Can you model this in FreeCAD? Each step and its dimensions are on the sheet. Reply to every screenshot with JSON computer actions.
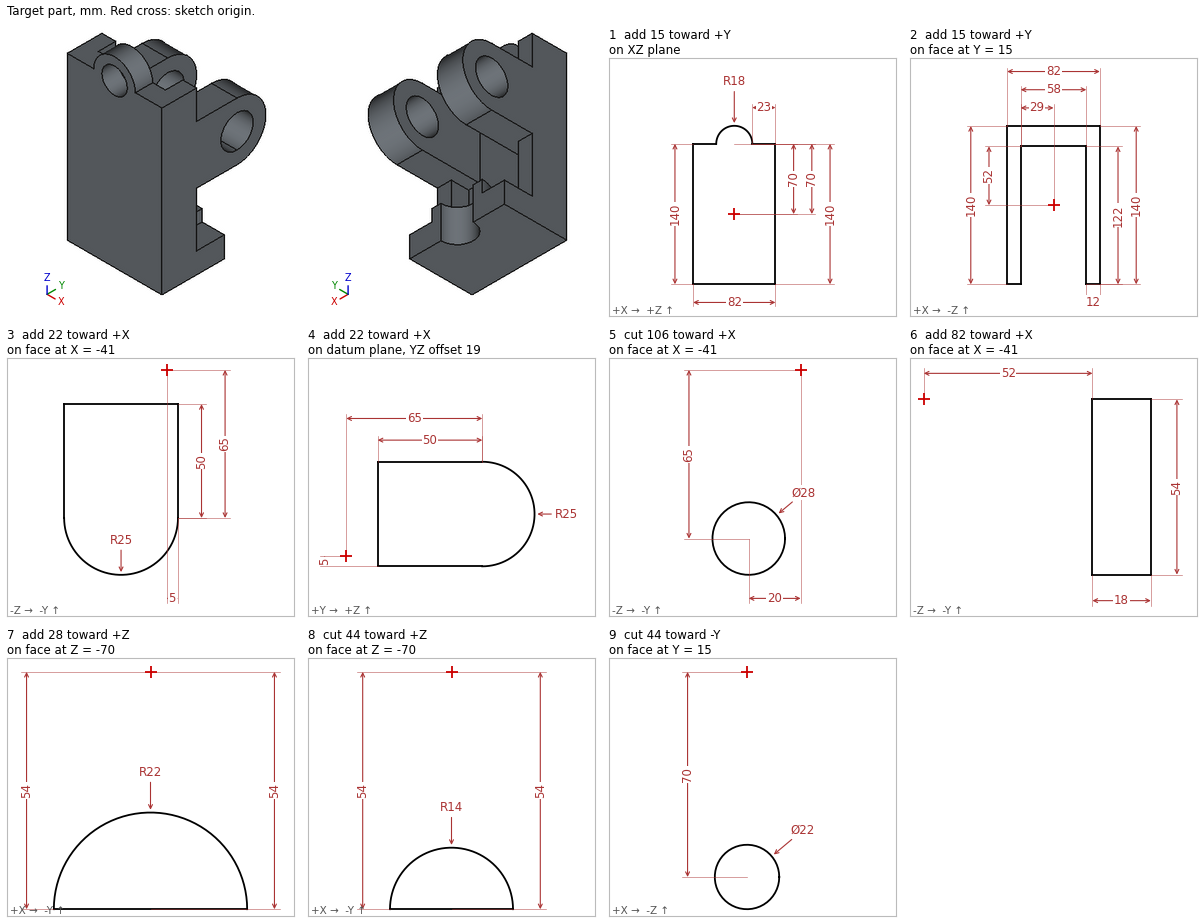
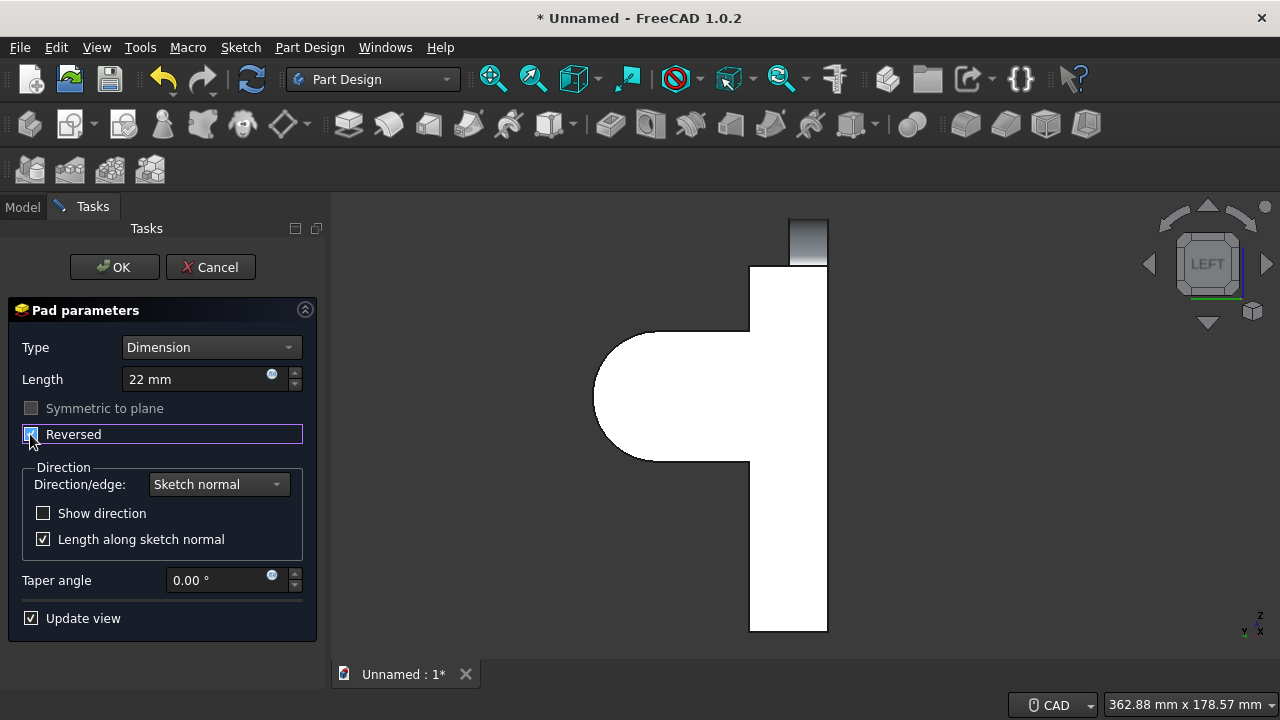
{"action": "left_click", "coordinate": [115, 267]}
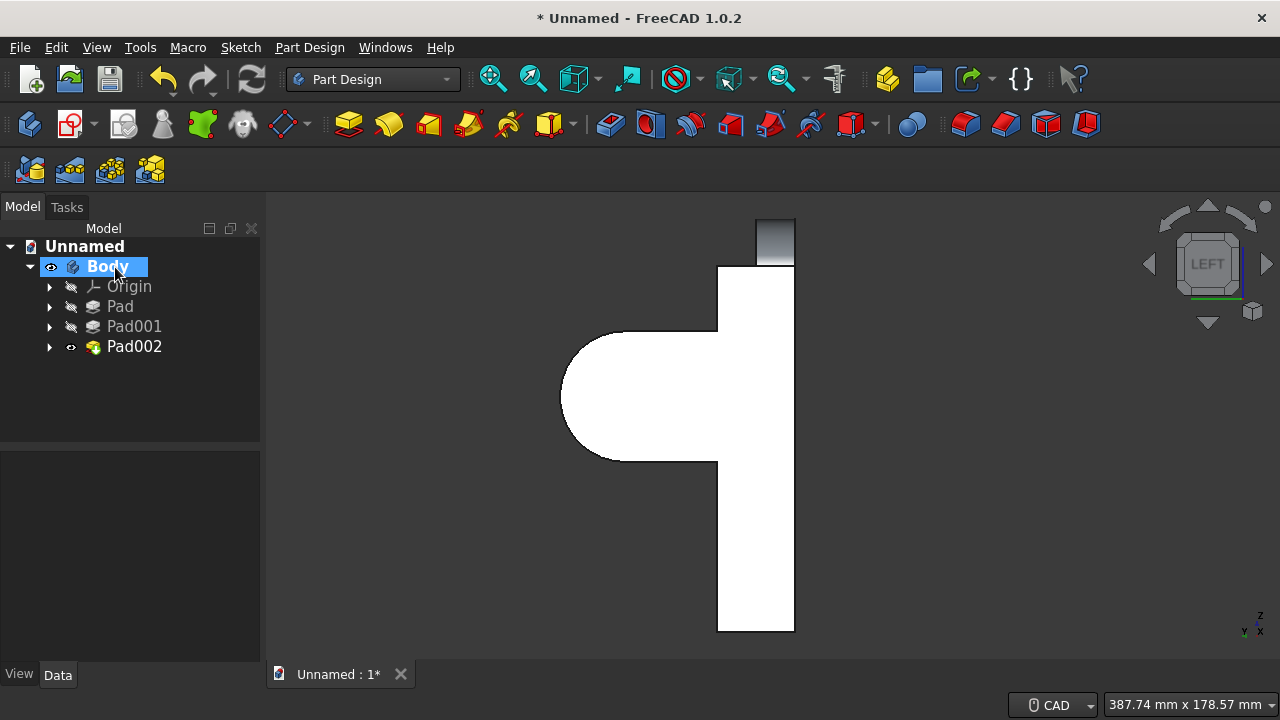
{"action": "left_click", "coordinate": [50, 287]}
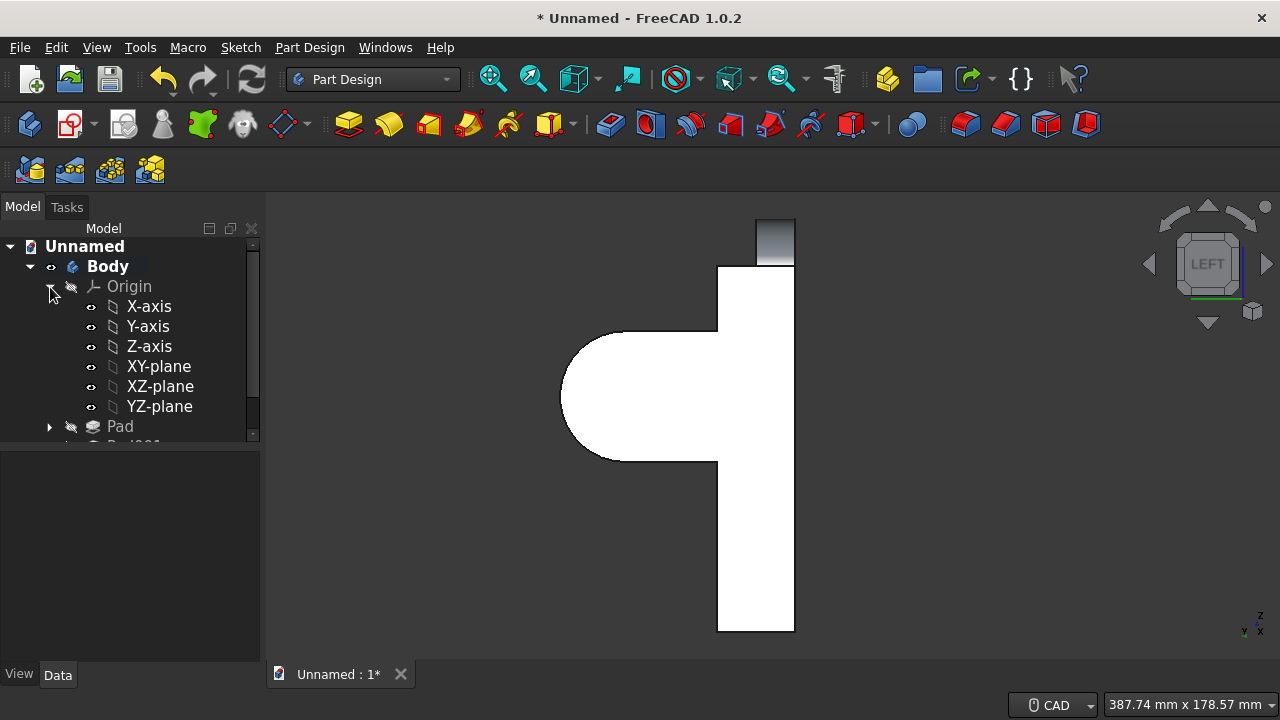
{"action": "left_click", "coordinate": [136, 407]}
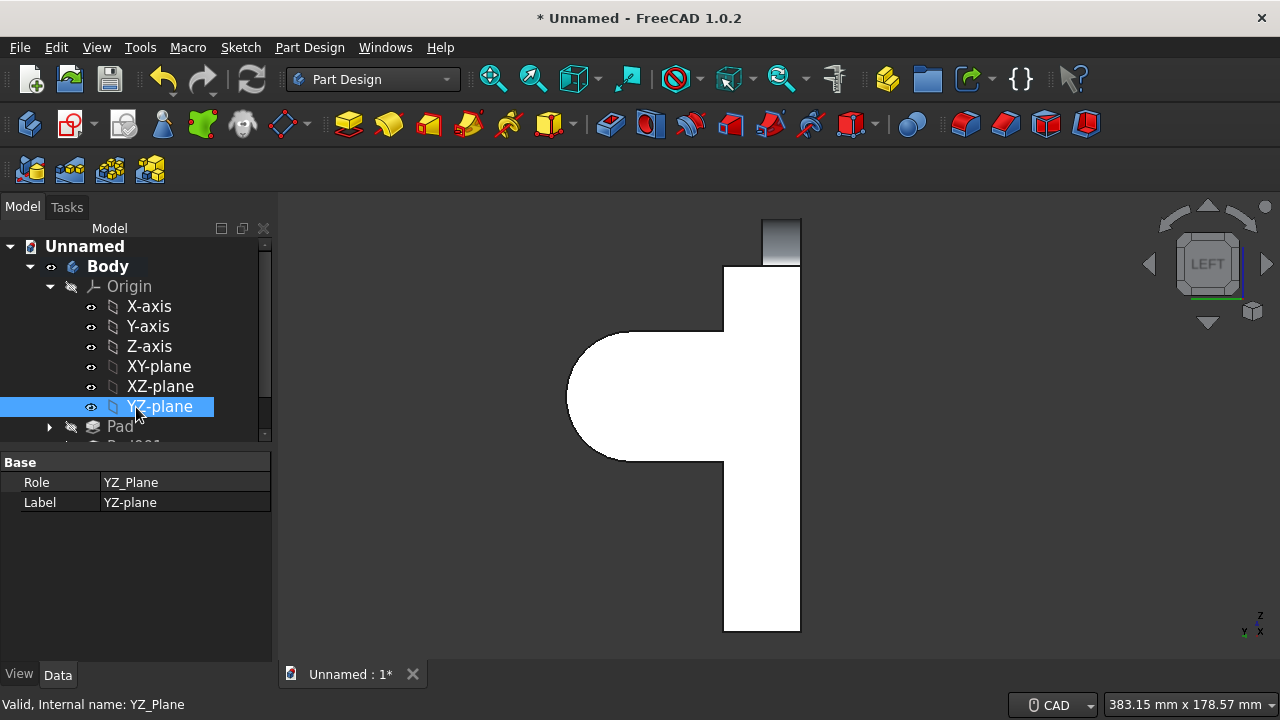
{"action": "left_click", "coordinate": [284, 124]}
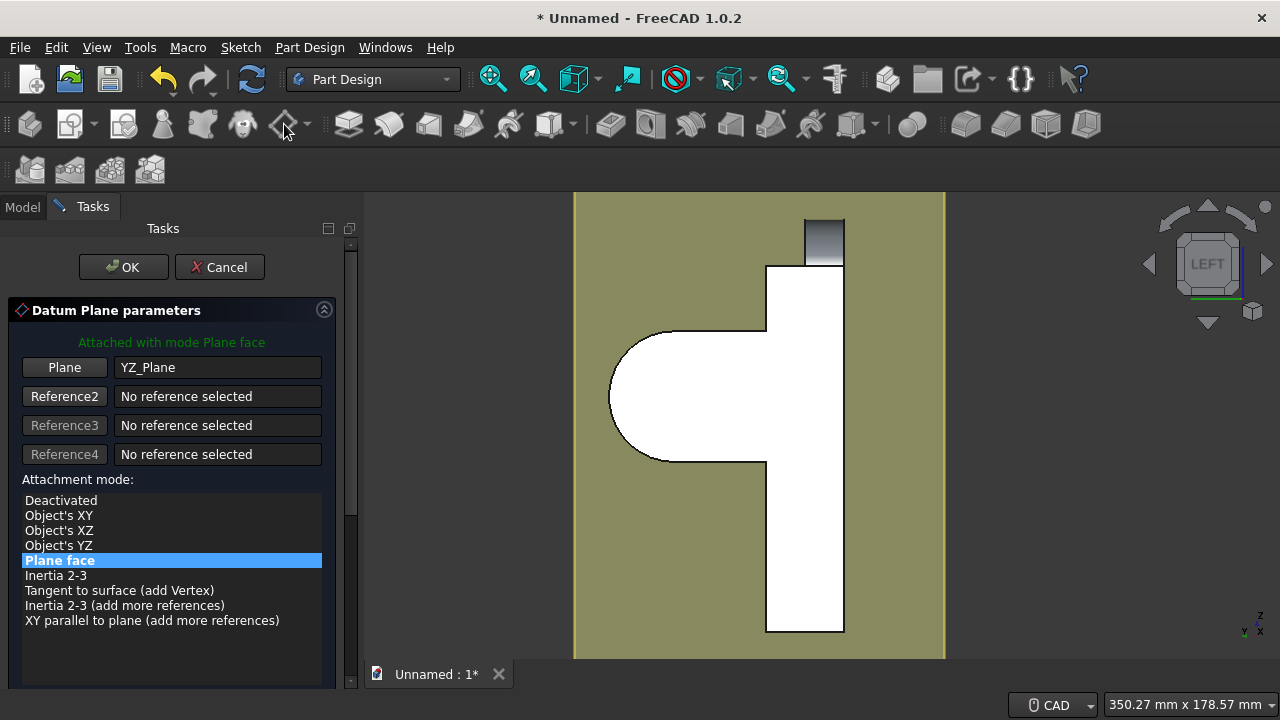
{"action": "scroll", "coordinate": [351, 463], "scroll_direction": "down", "scroll_amount": 3}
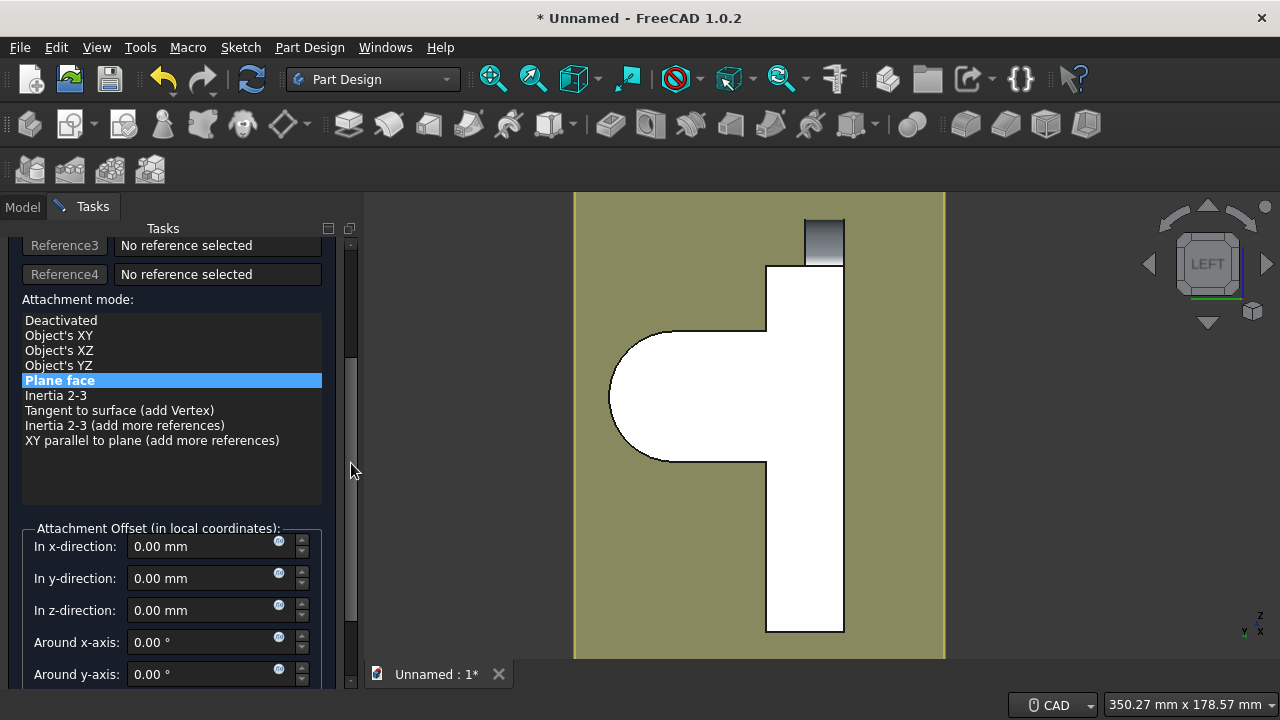
{"action": "triple_click", "coordinate": [210, 610]}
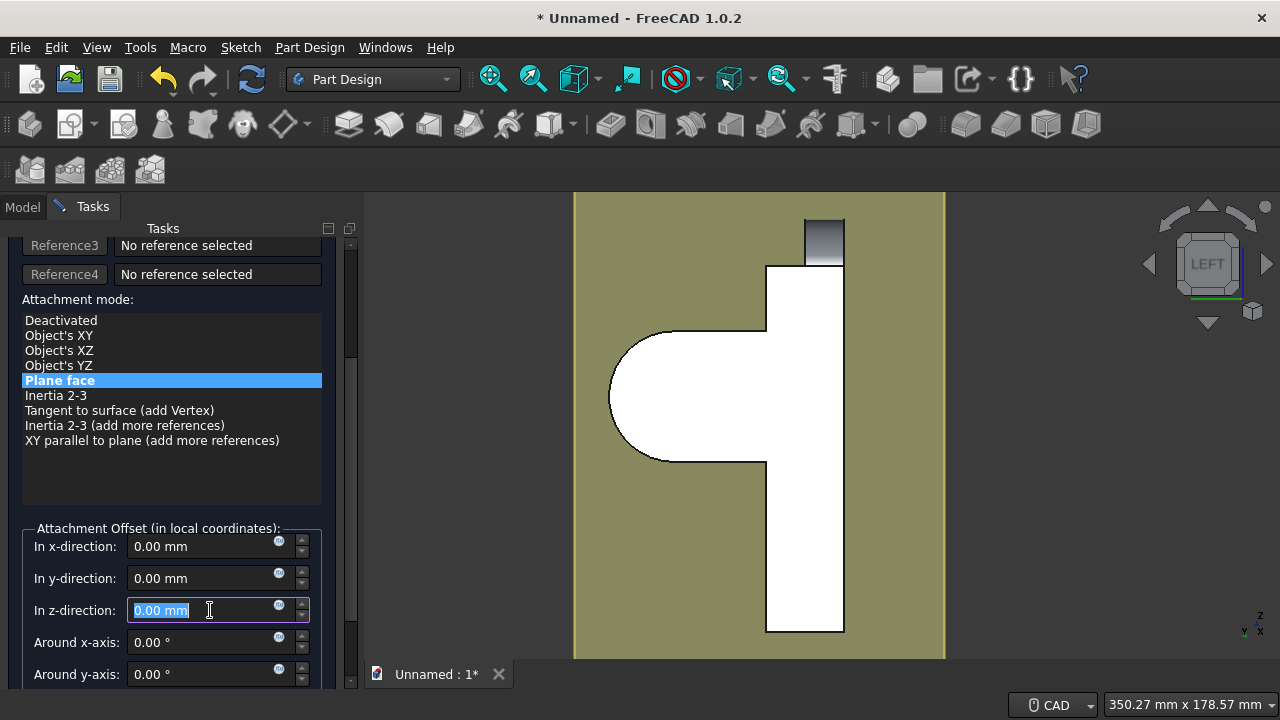
{"action": "type", "text": "19"}
{"action": "key", "text": "Tab"}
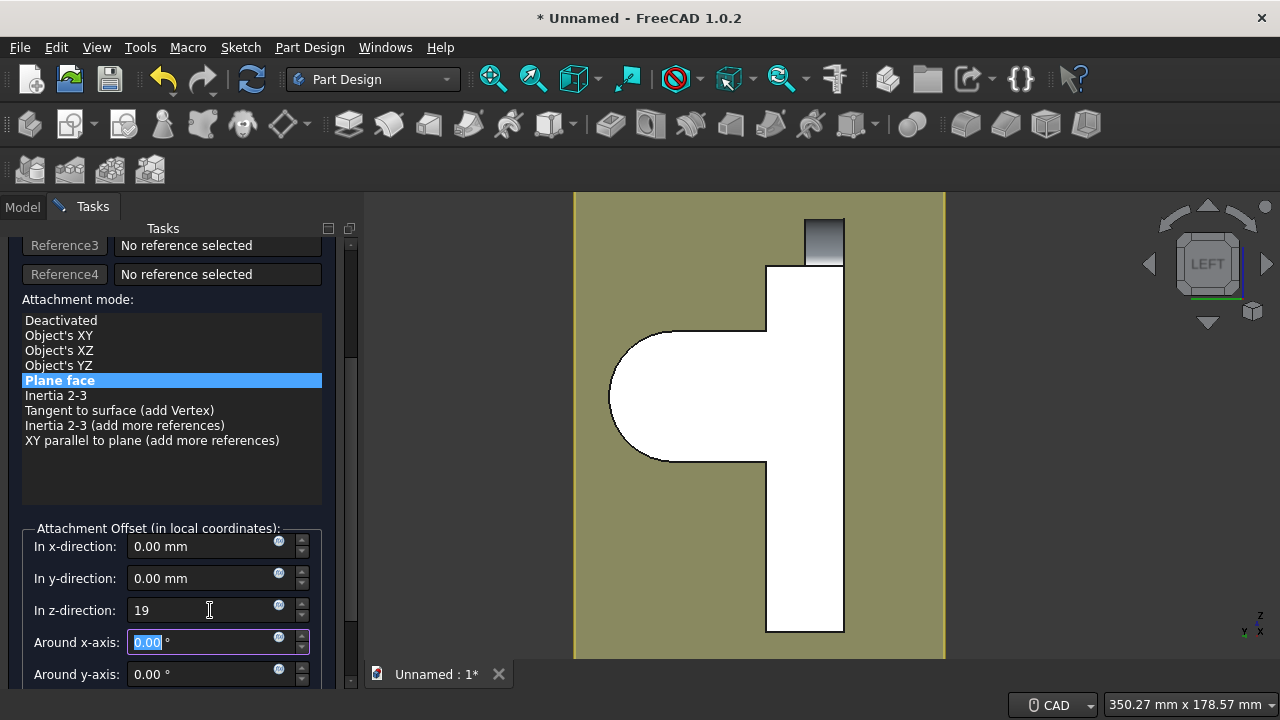
{"action": "scroll", "coordinate": [351, 463], "scroll_direction": "up", "scroll_amount": 4}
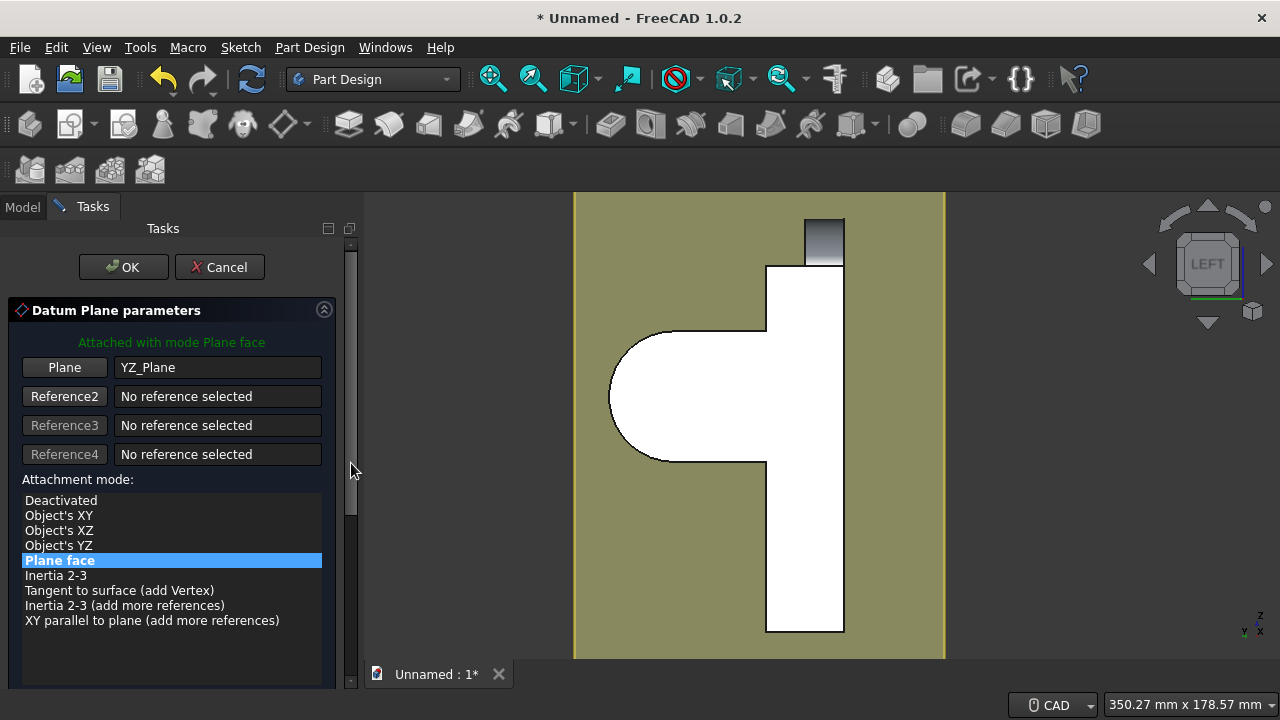
{"action": "left_click", "coordinate": [124, 267]}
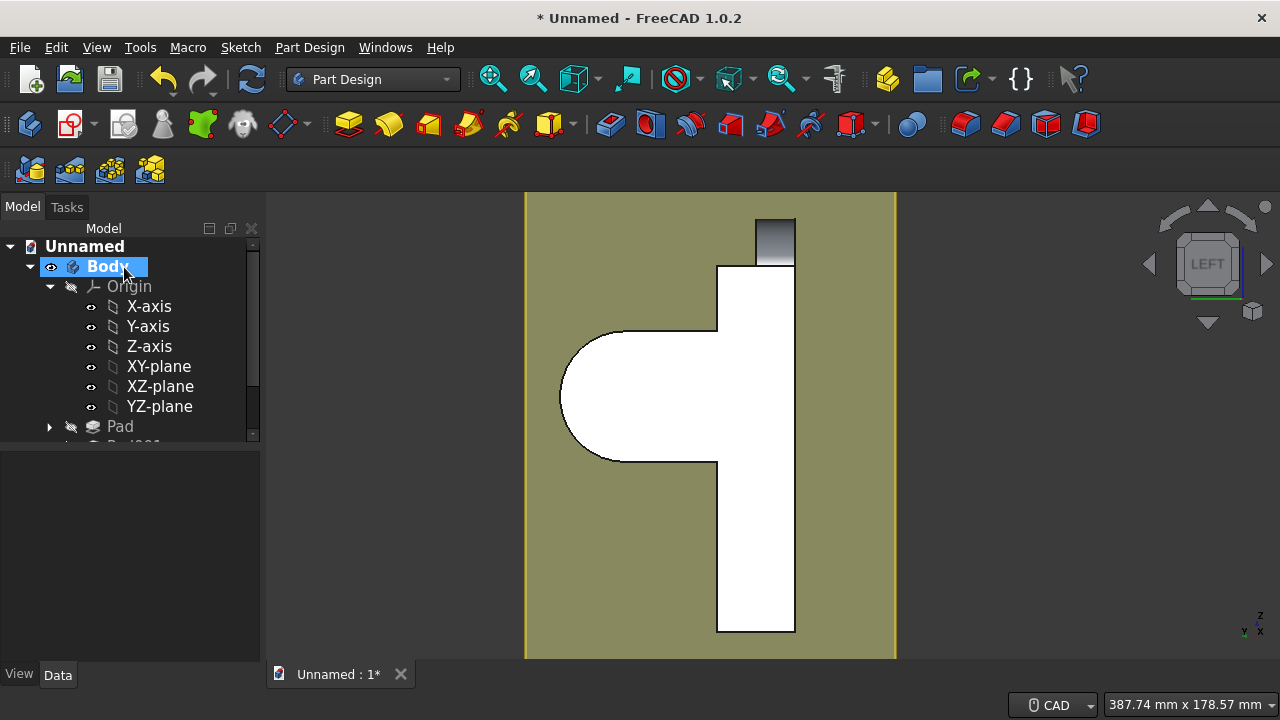
{"action": "scroll", "coordinate": [100, 342], "scroll_direction": "down", "scroll_amount": 3}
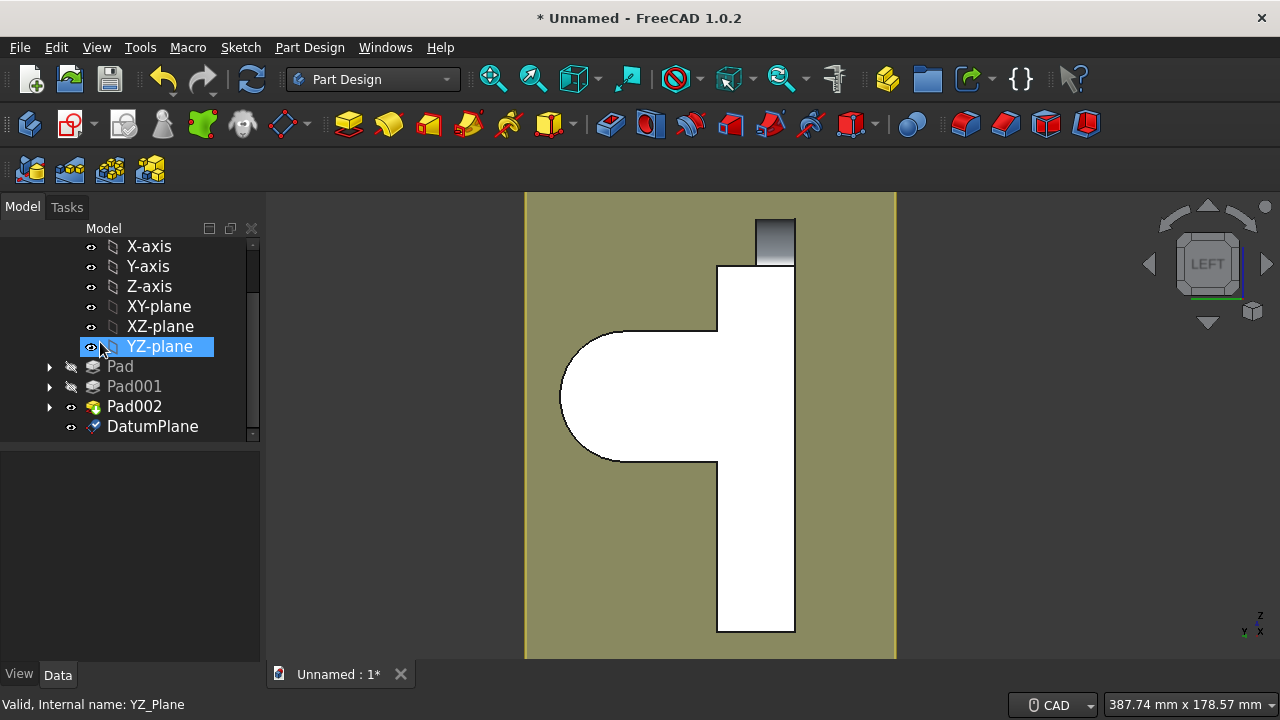
{"action": "left_click", "coordinate": [116, 427]}